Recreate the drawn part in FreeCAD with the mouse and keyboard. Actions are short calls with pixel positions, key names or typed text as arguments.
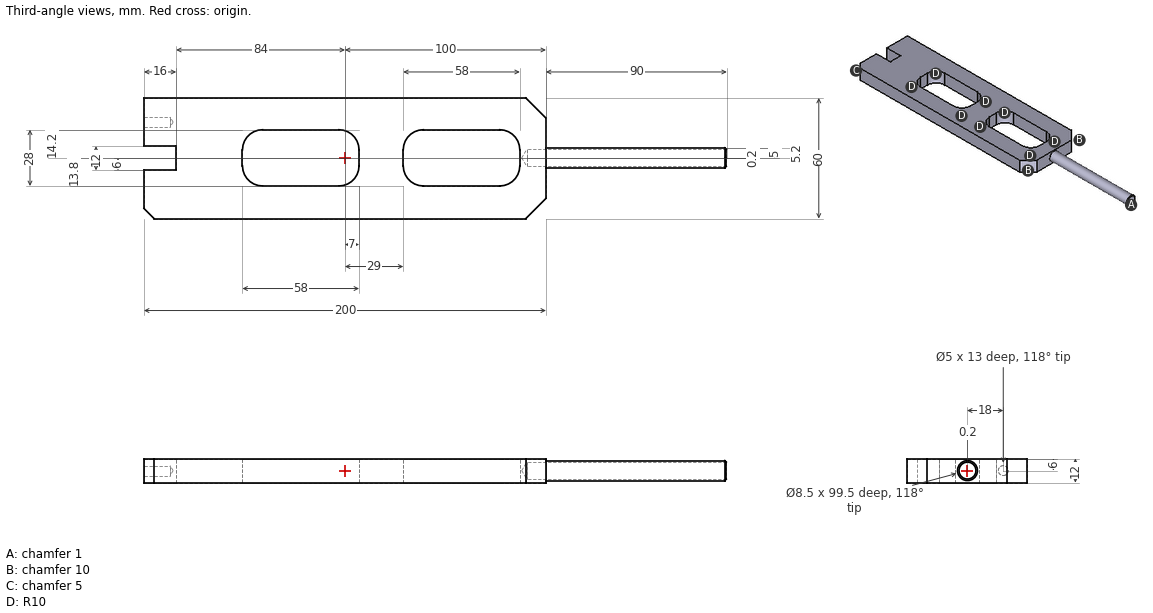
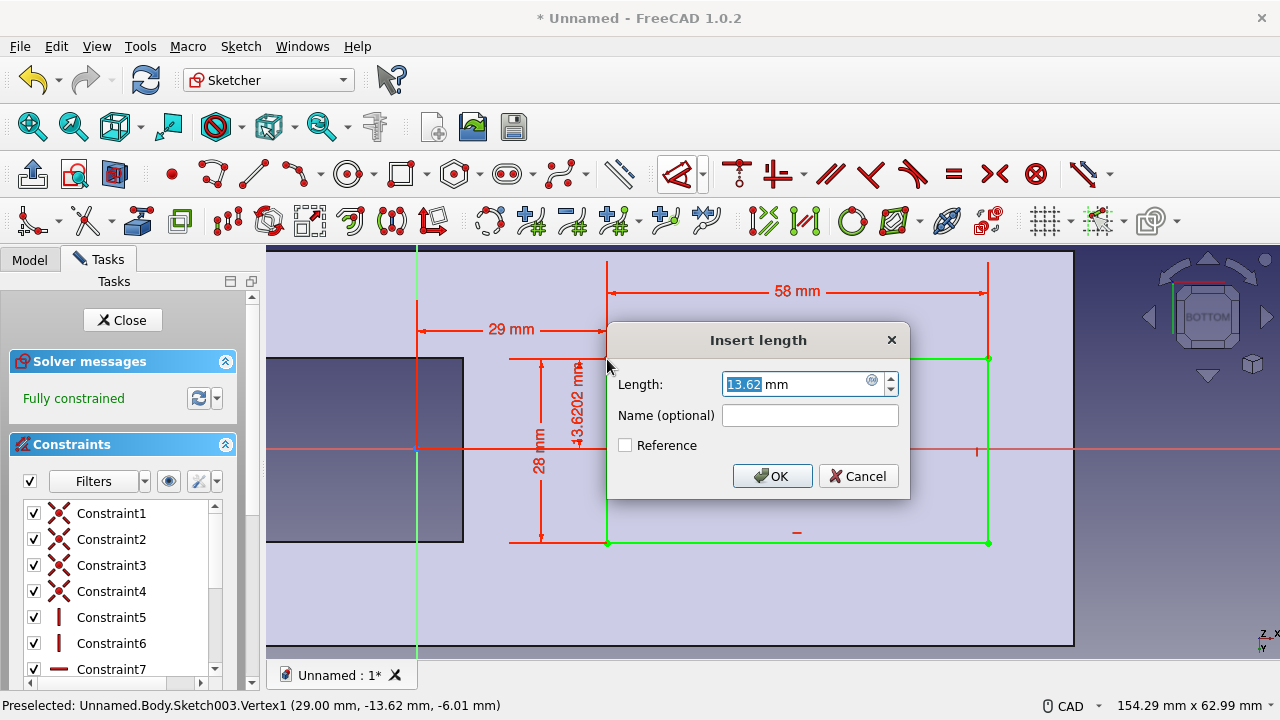
text(13.8)
key(Return)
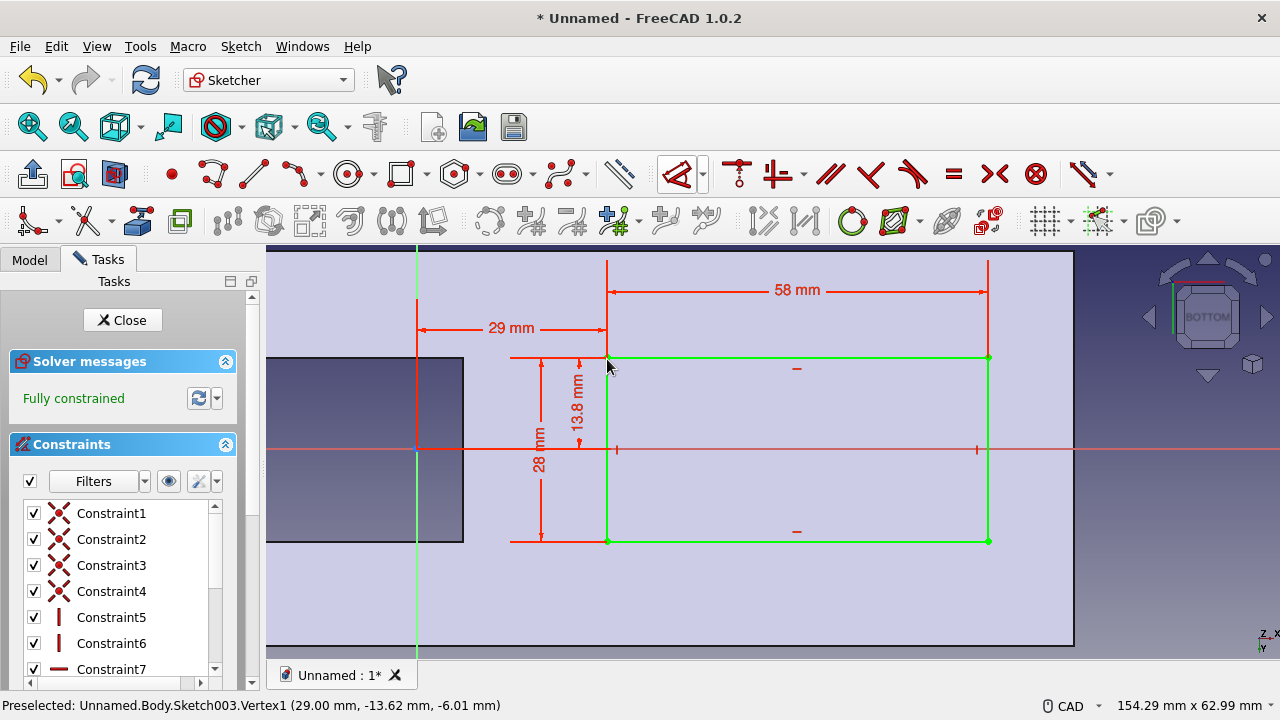
click(123, 320)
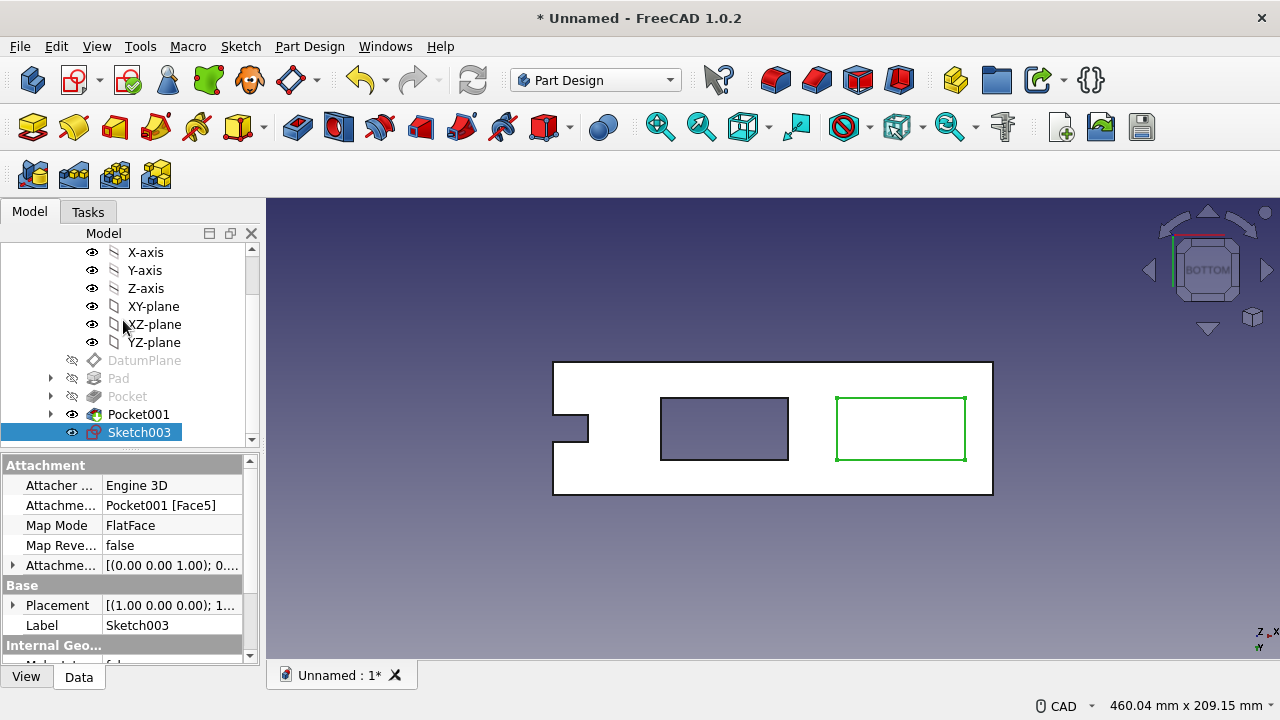
click(298, 128)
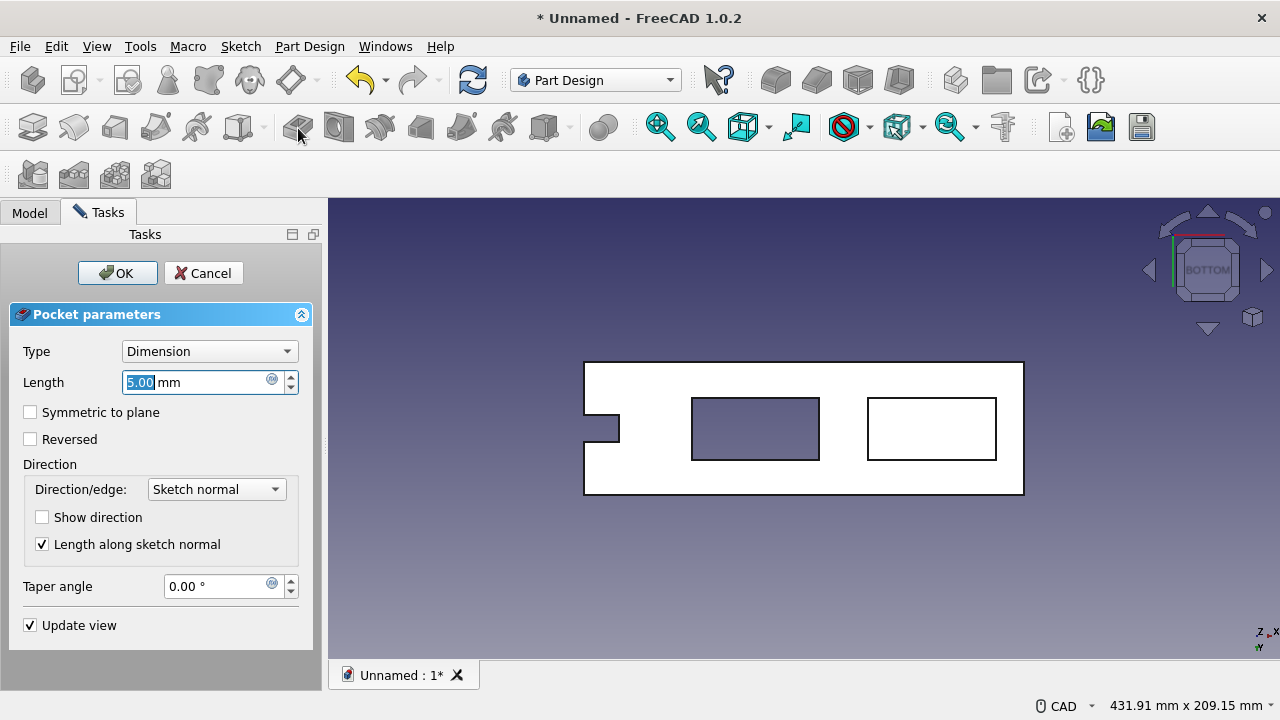
click(210, 352)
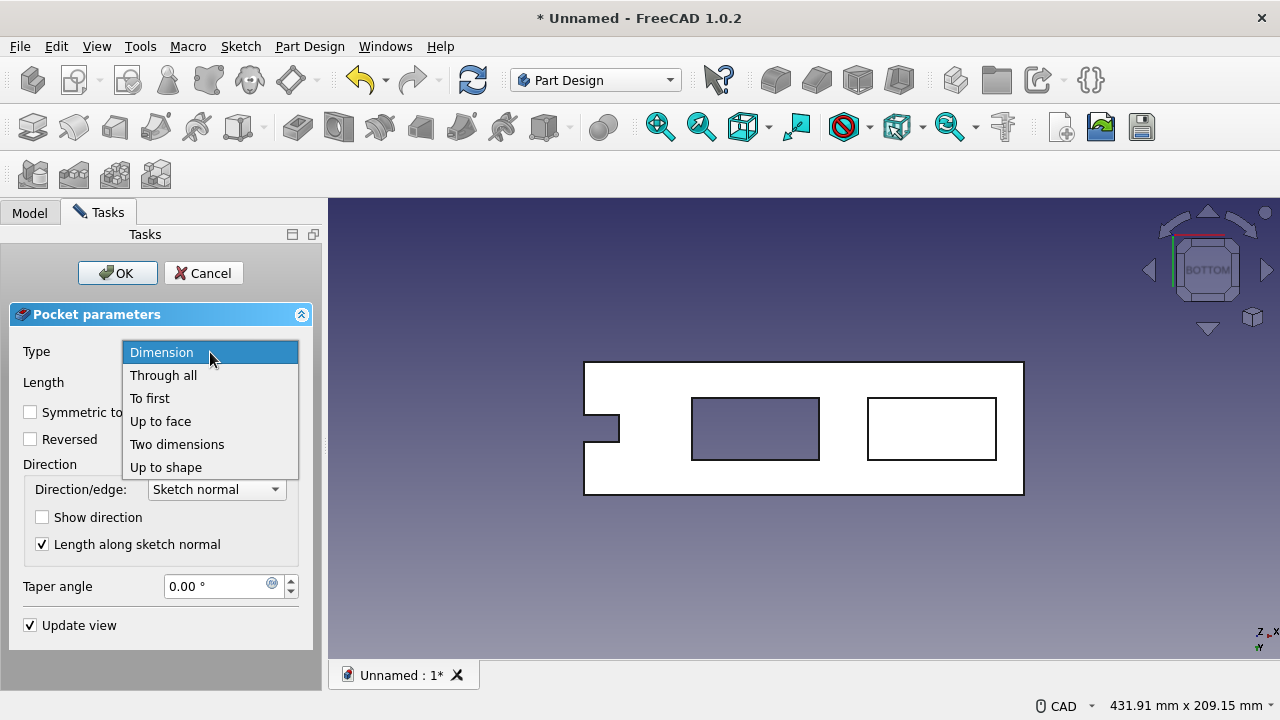
click(208, 376)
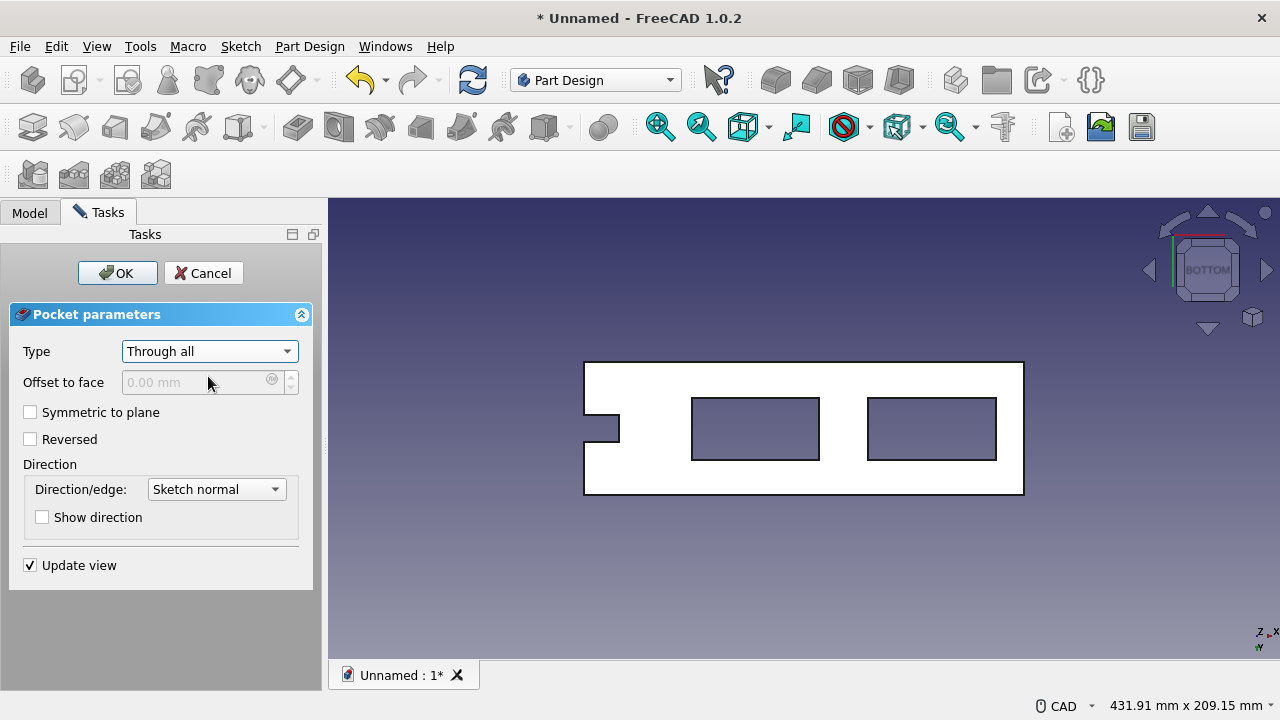
click(118, 273)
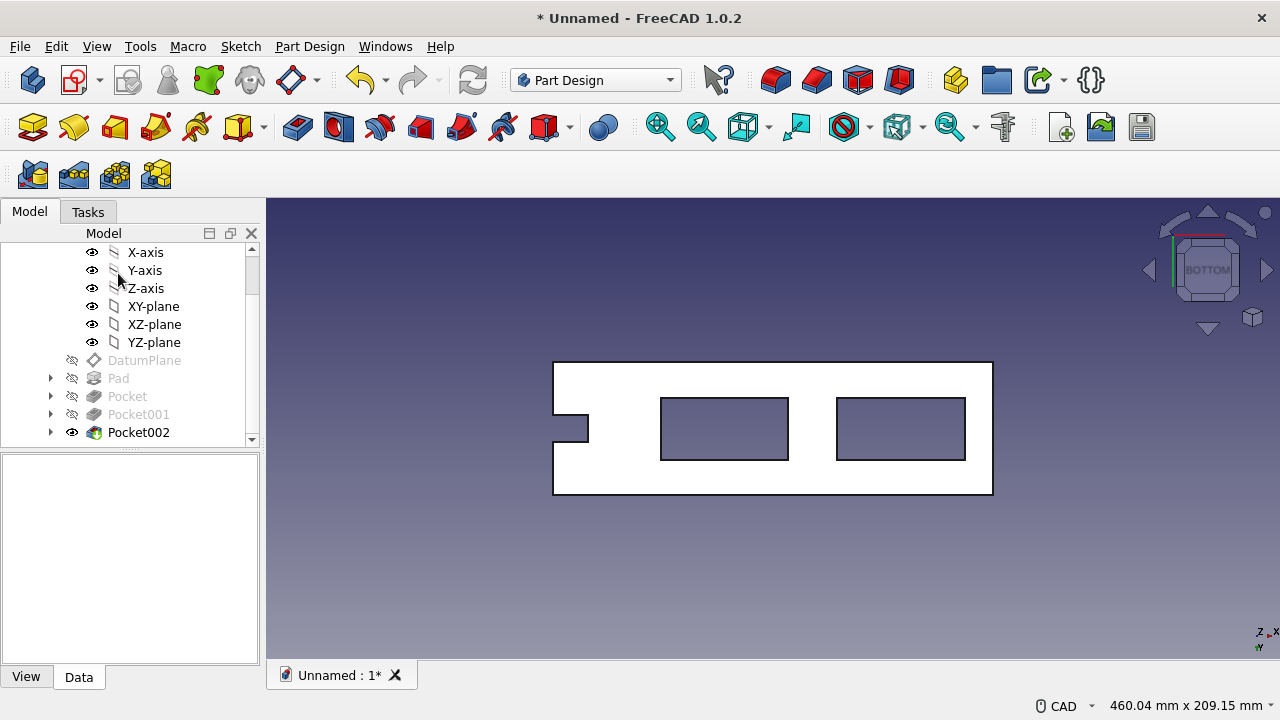
key(v)
key(f)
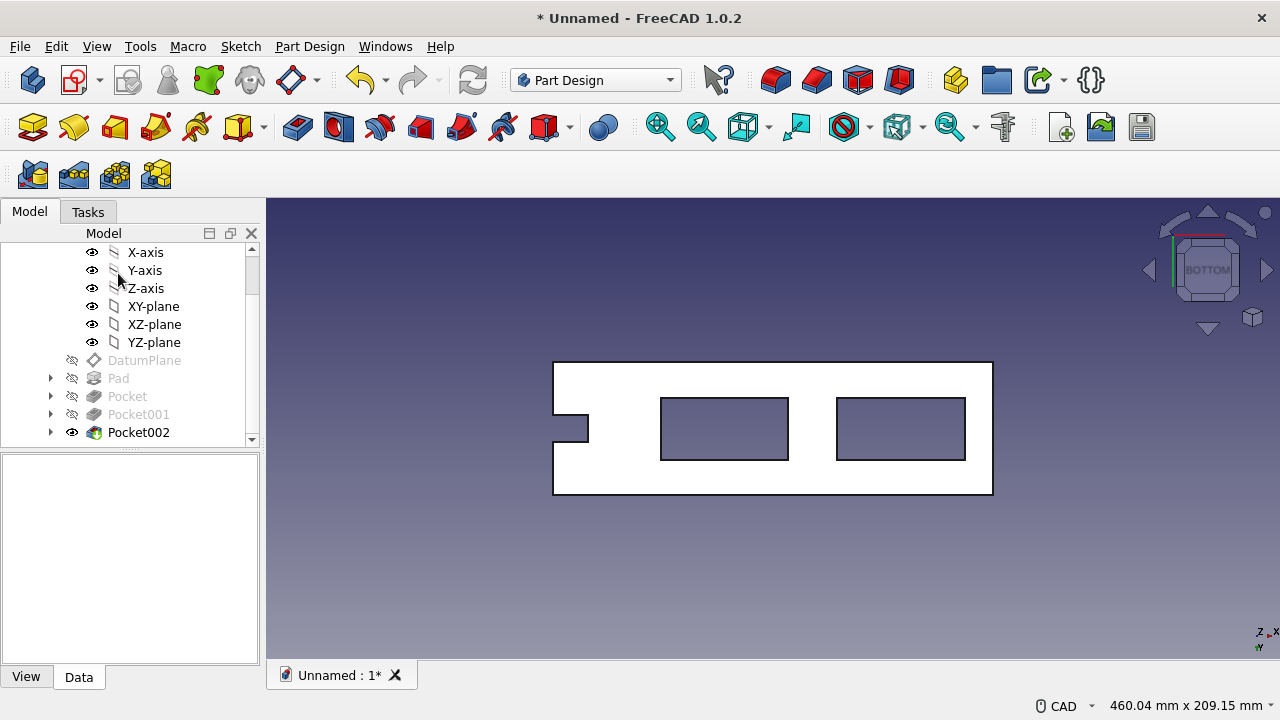
click(74, 80)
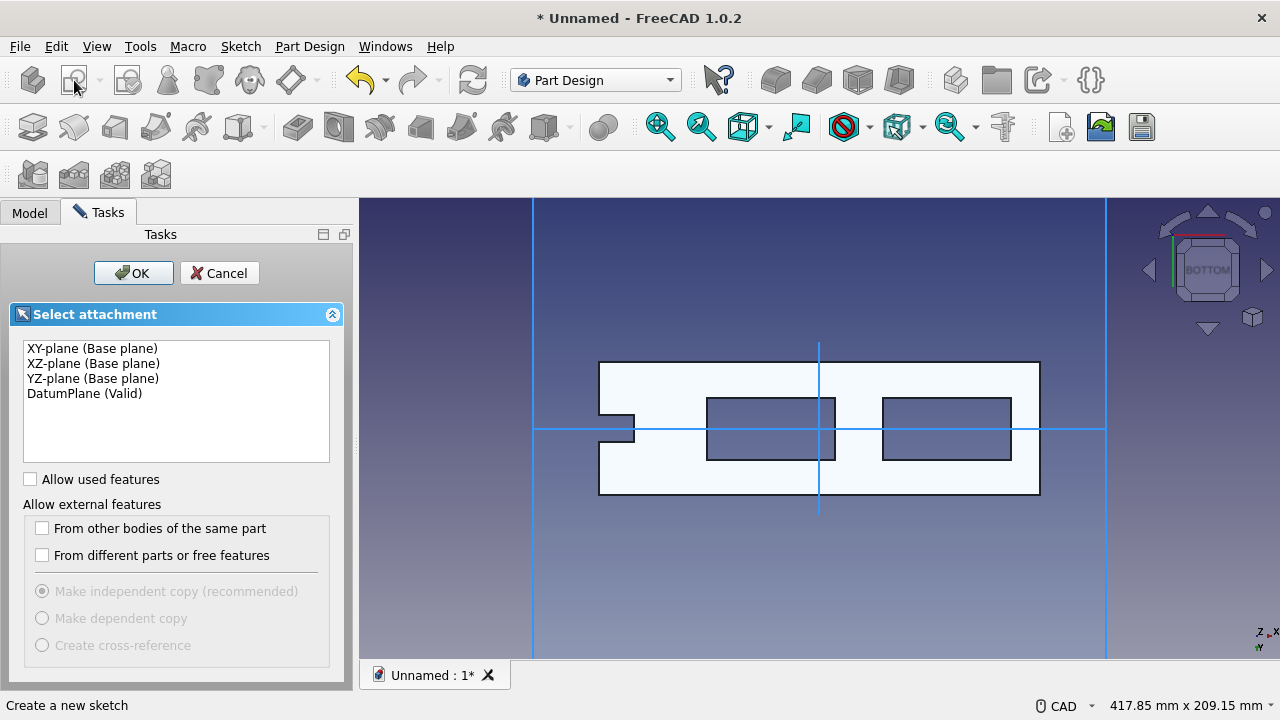
click(84, 348)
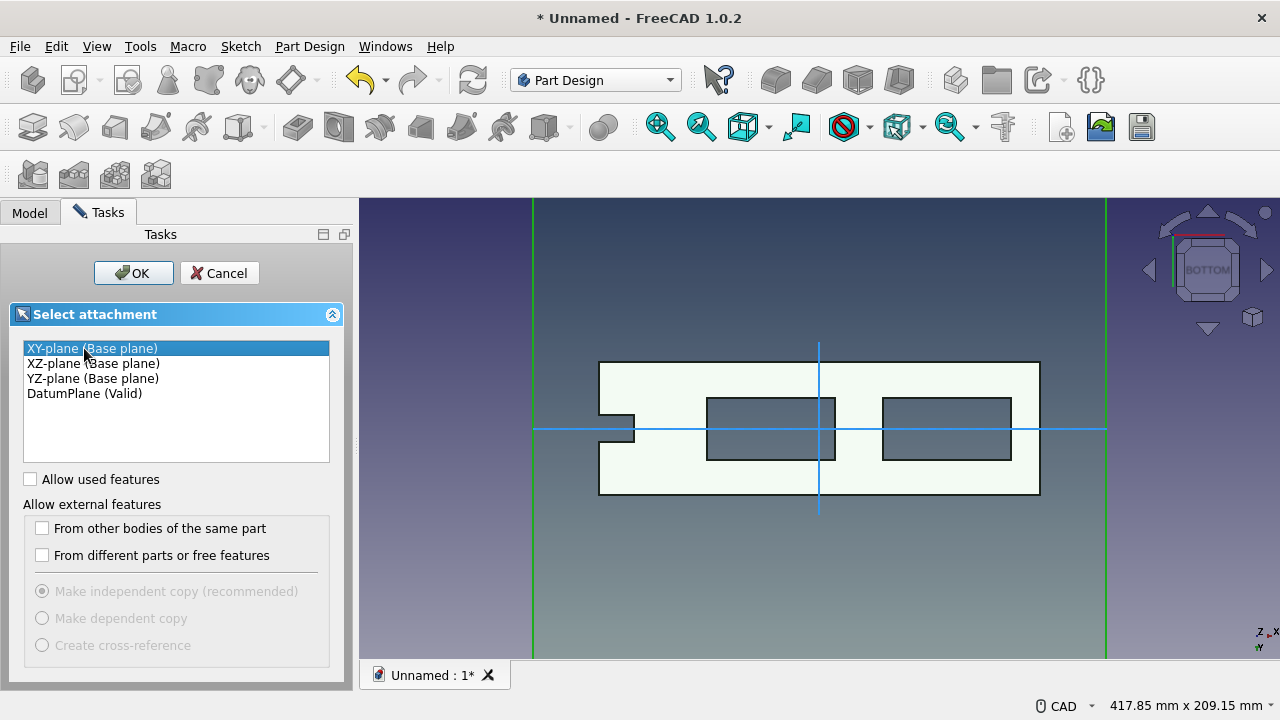
click(134, 273)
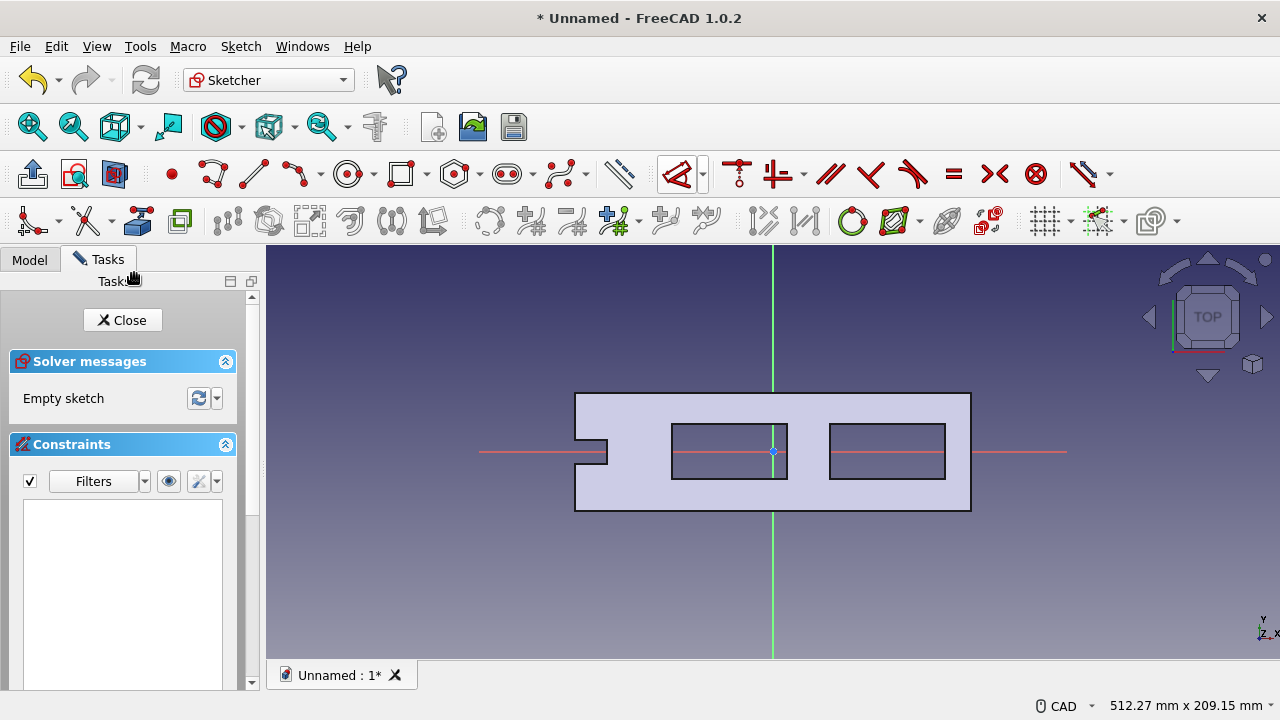
click(115, 174)